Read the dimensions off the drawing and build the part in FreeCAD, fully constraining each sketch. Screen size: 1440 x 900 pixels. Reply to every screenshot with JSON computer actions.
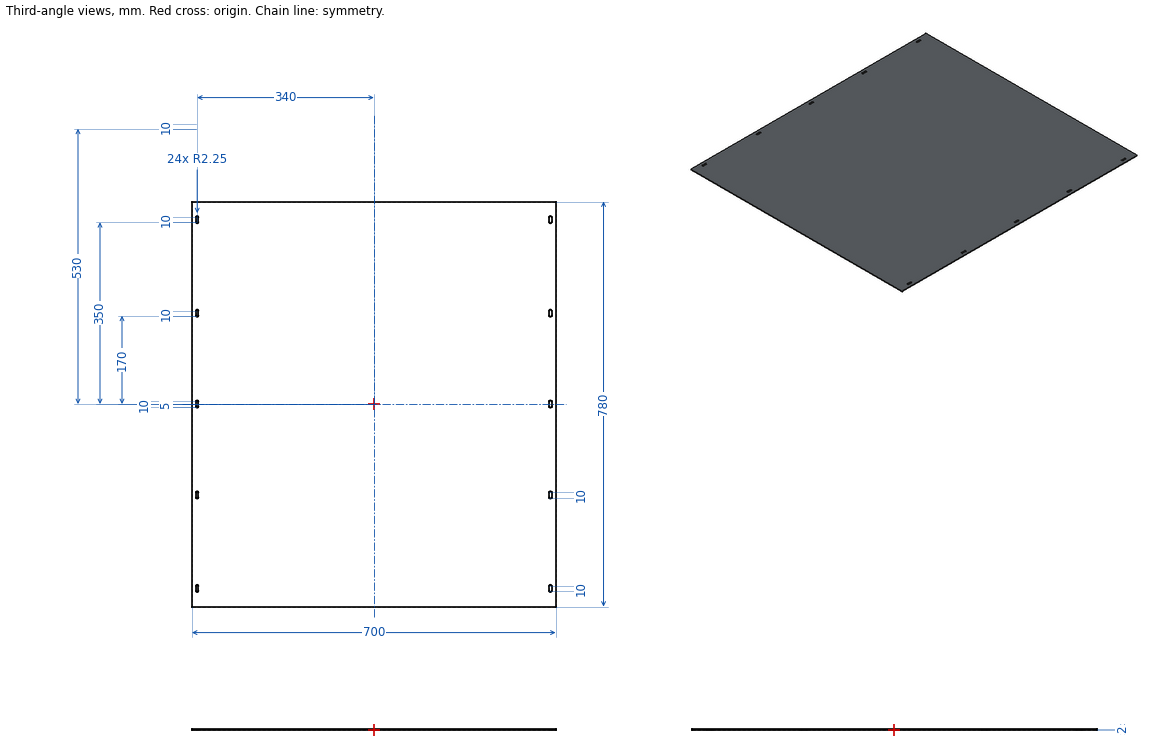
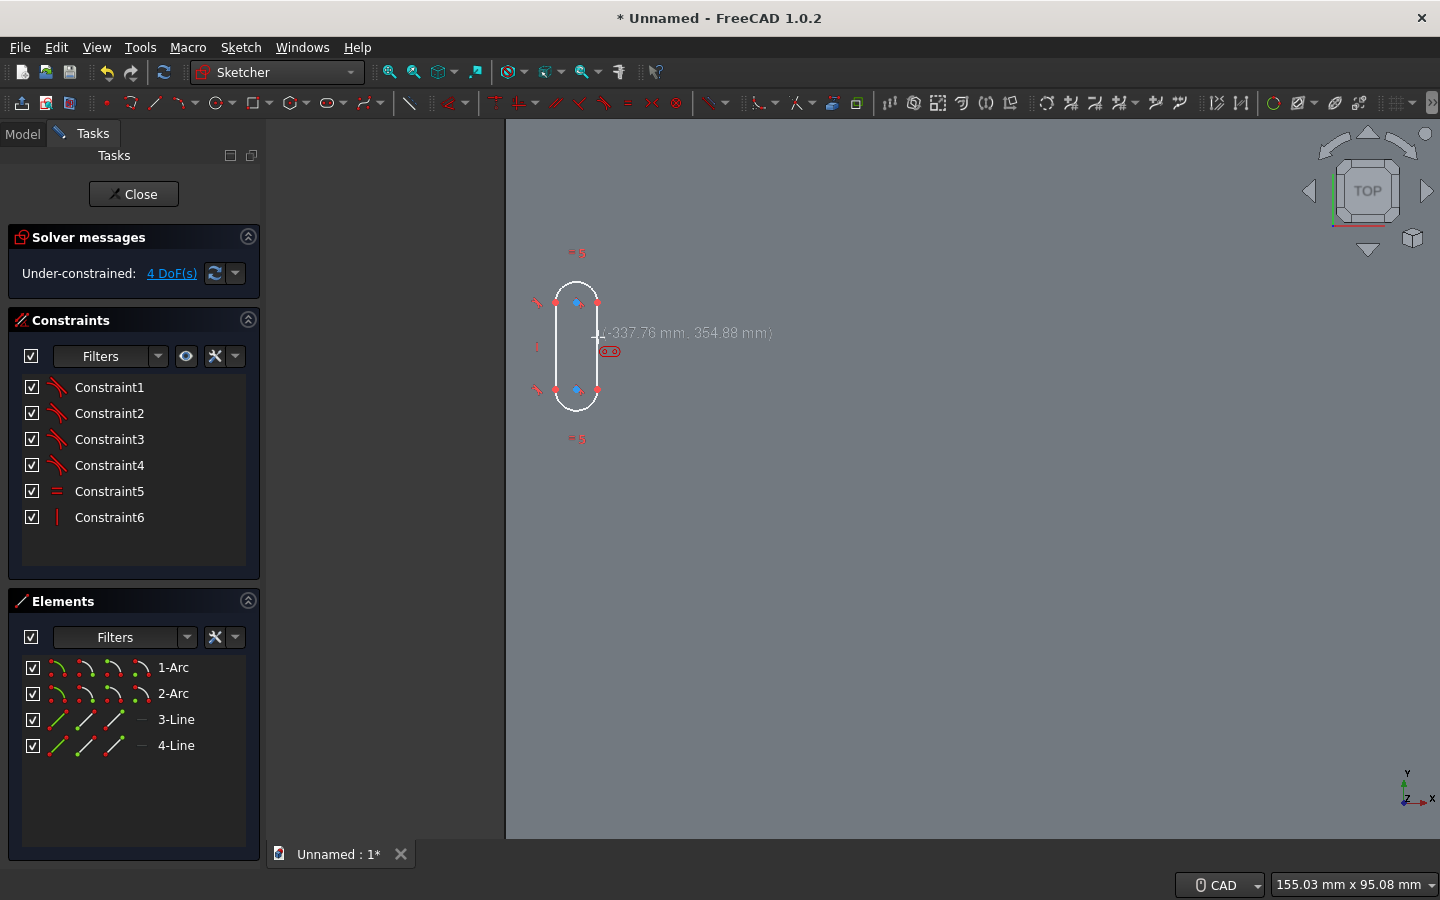
{"action": "scroll", "coordinate": [594, 329], "scroll_direction": "down", "scroll_amount": 13}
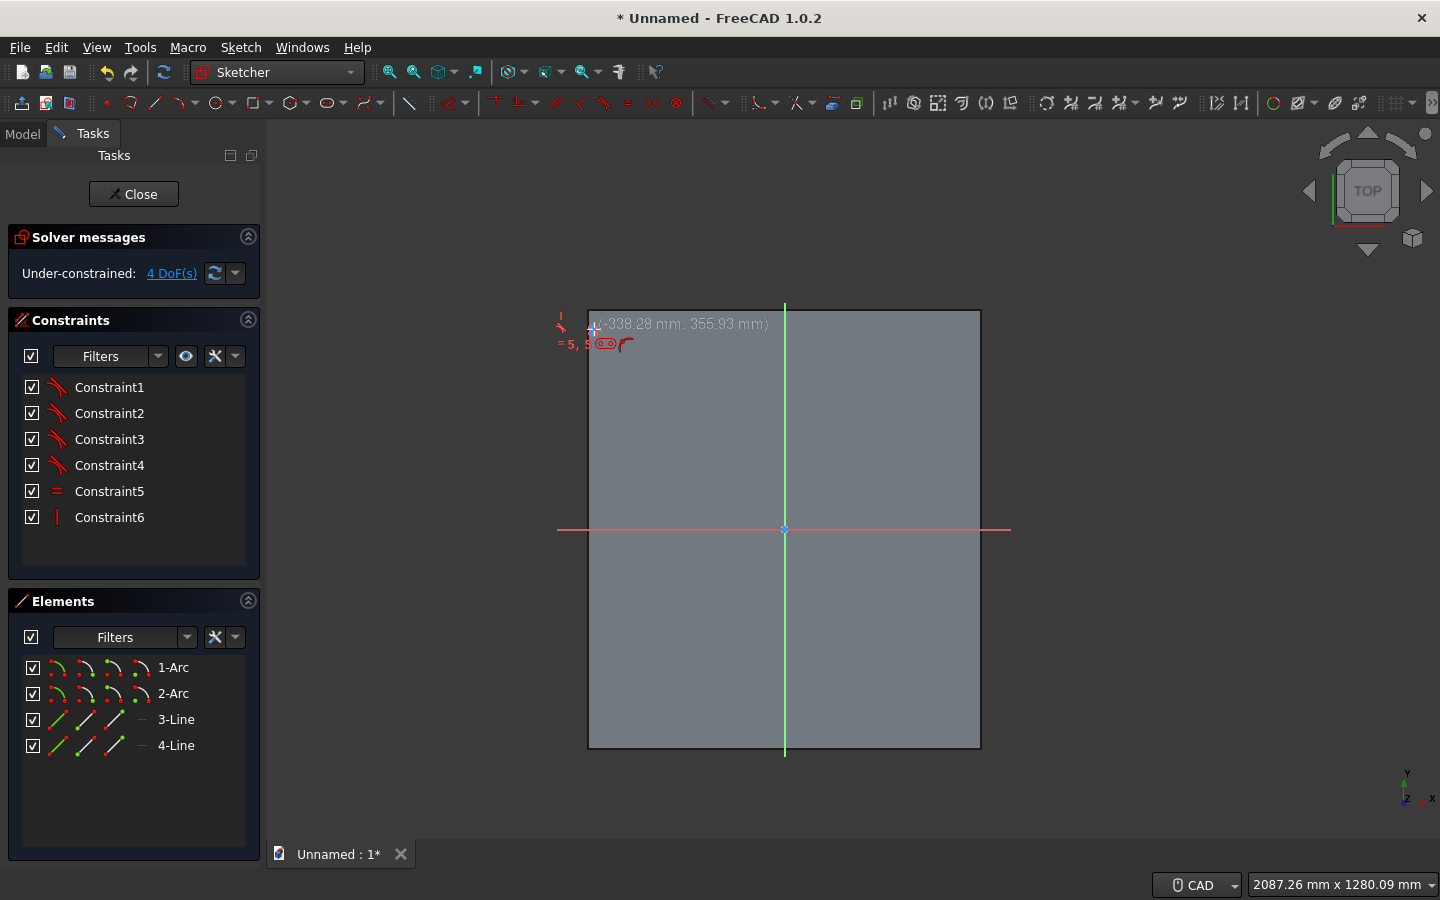
{"action": "scroll", "coordinate": [976, 333], "scroll_direction": "up", "scroll_amount": 15}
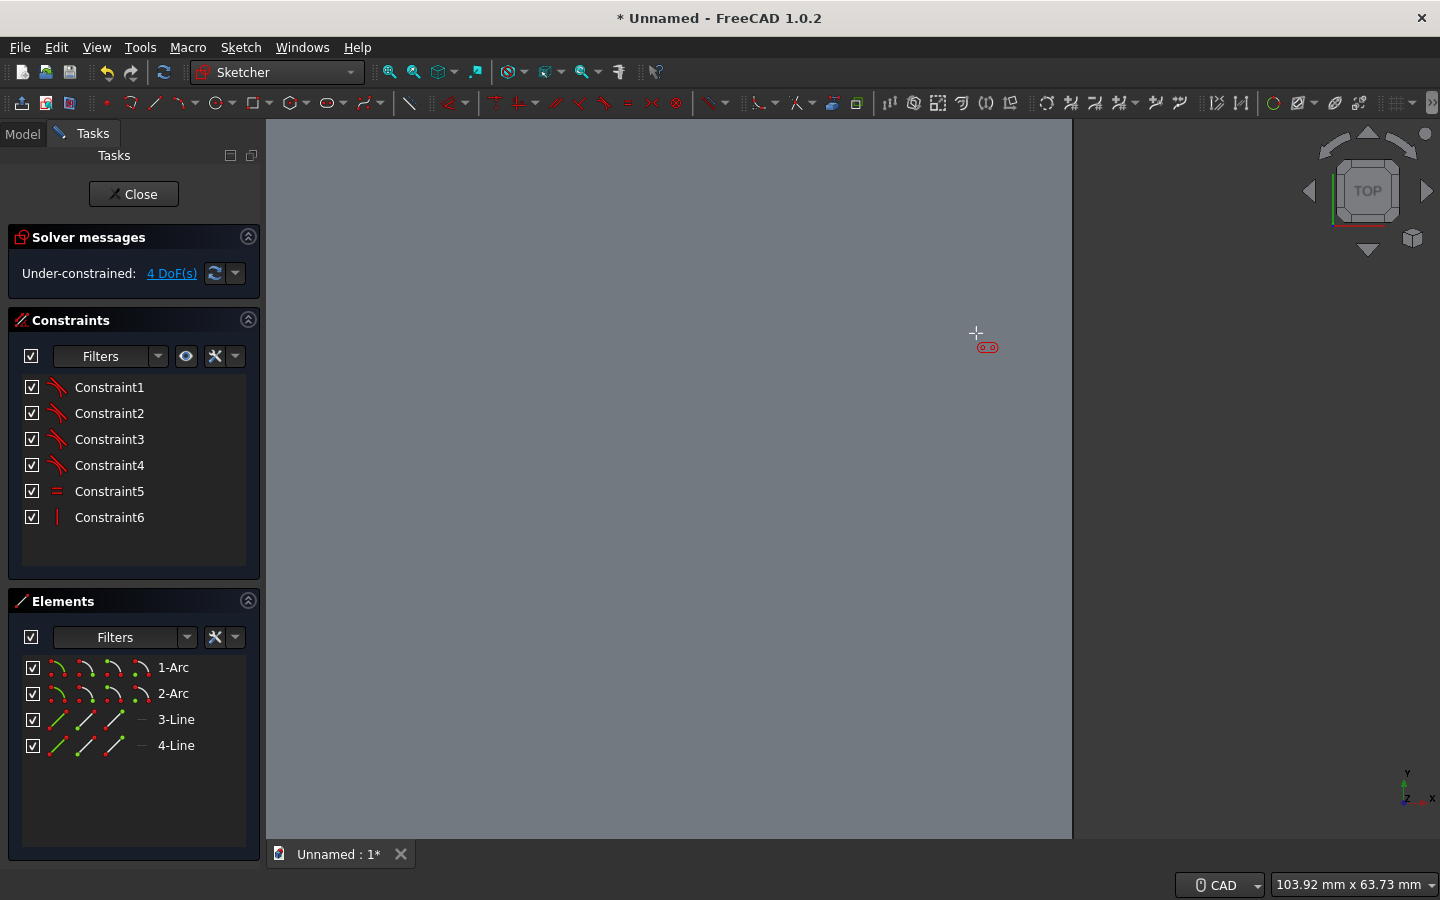
{"action": "scroll", "coordinate": [977, 333], "scroll_direction": "down", "scroll_amount": 15}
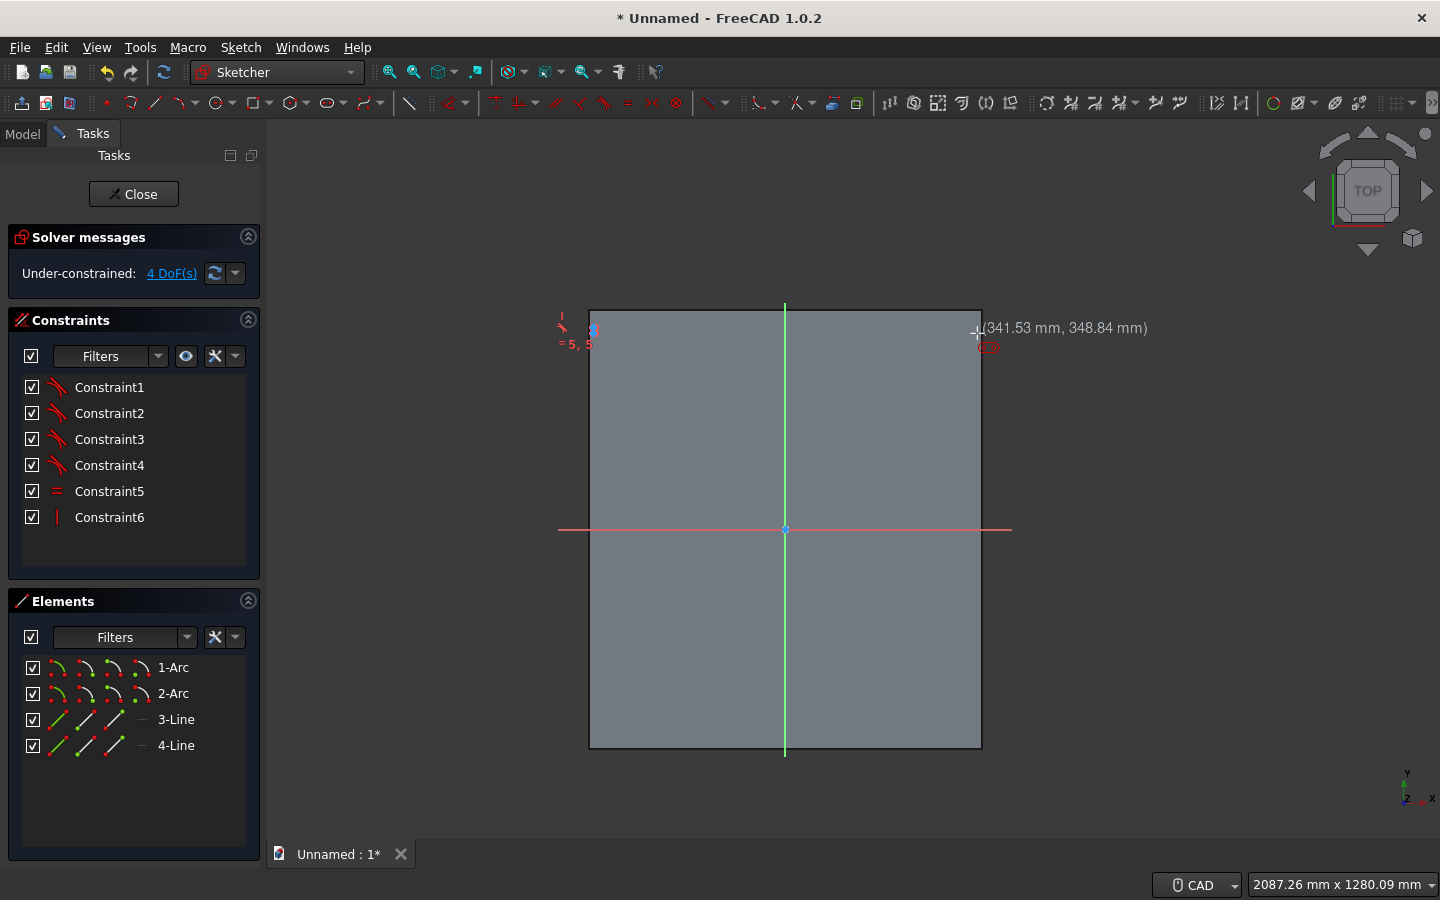
{"action": "left_click", "coordinate": [977, 333]}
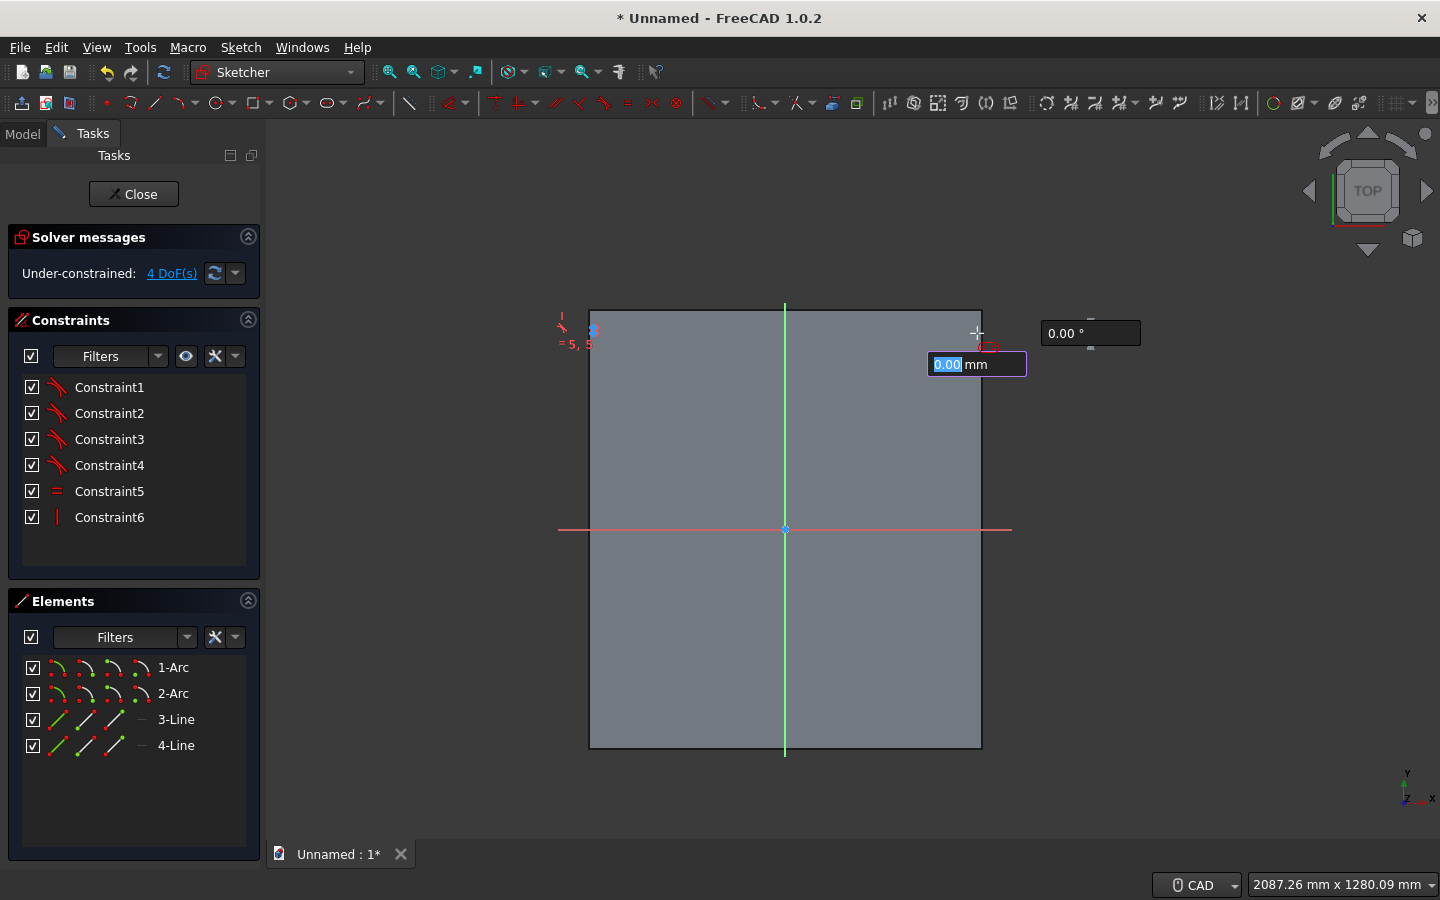
{"action": "scroll", "coordinate": [977, 327], "scroll_direction": "up", "scroll_amount": 6}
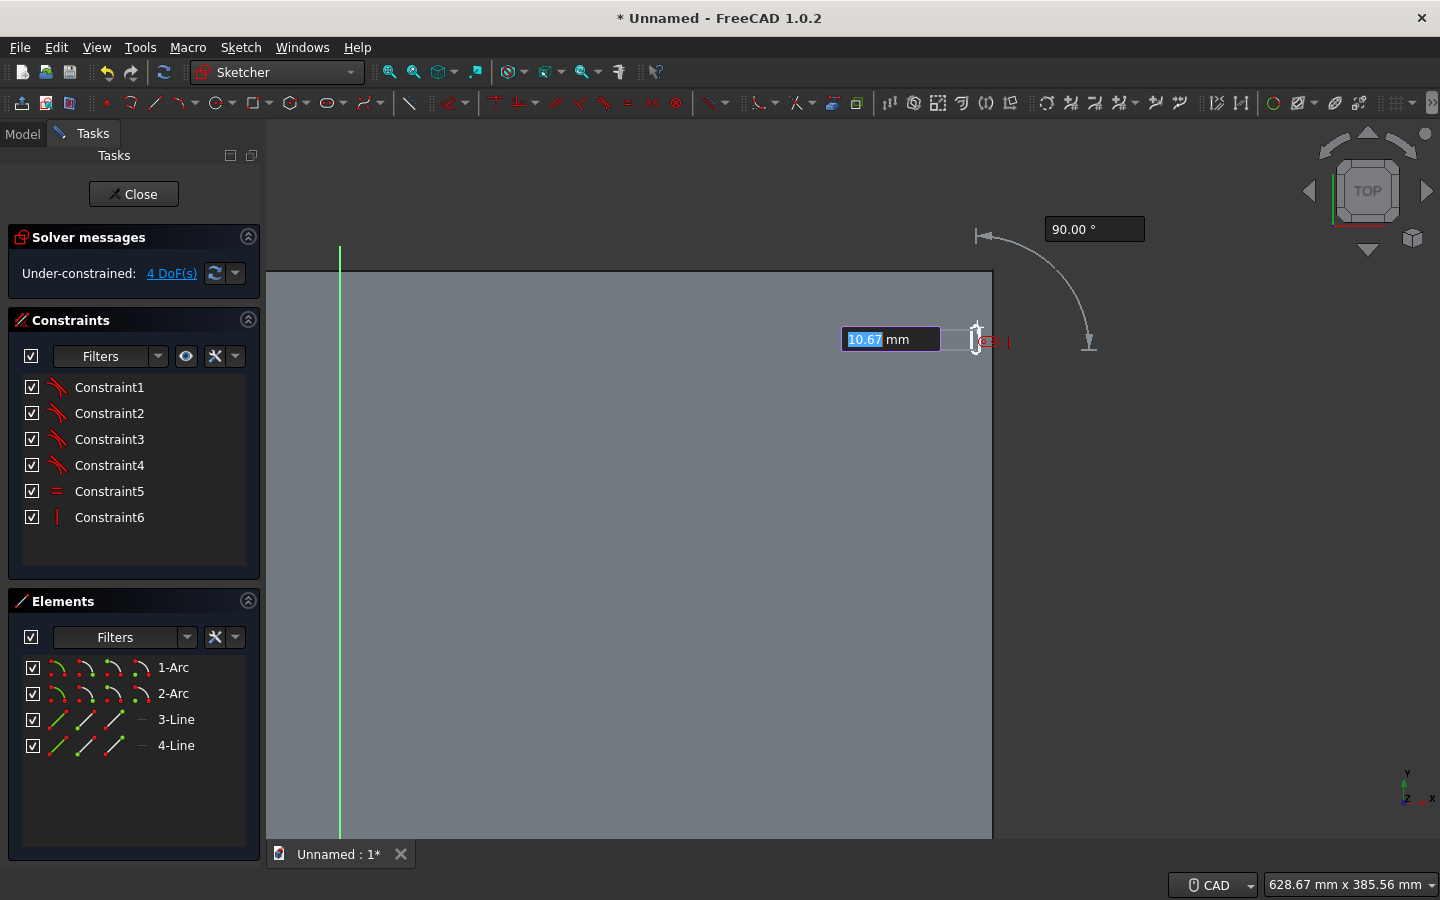
{"action": "left_click", "coordinate": [976, 327]}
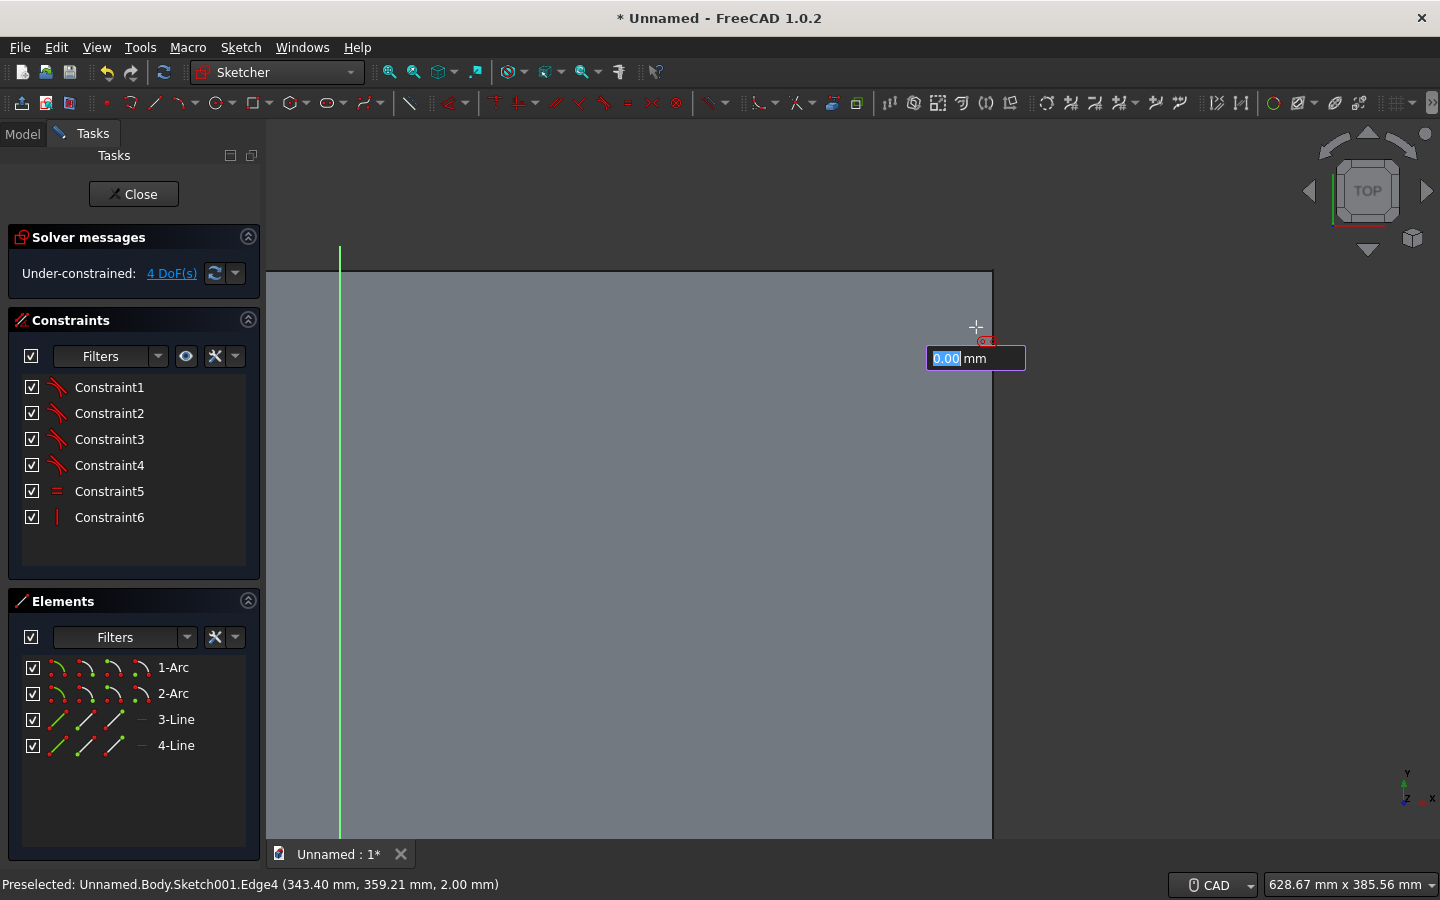
{"action": "scroll", "coordinate": [970, 336], "scroll_direction": "up", "scroll_amount": 7}